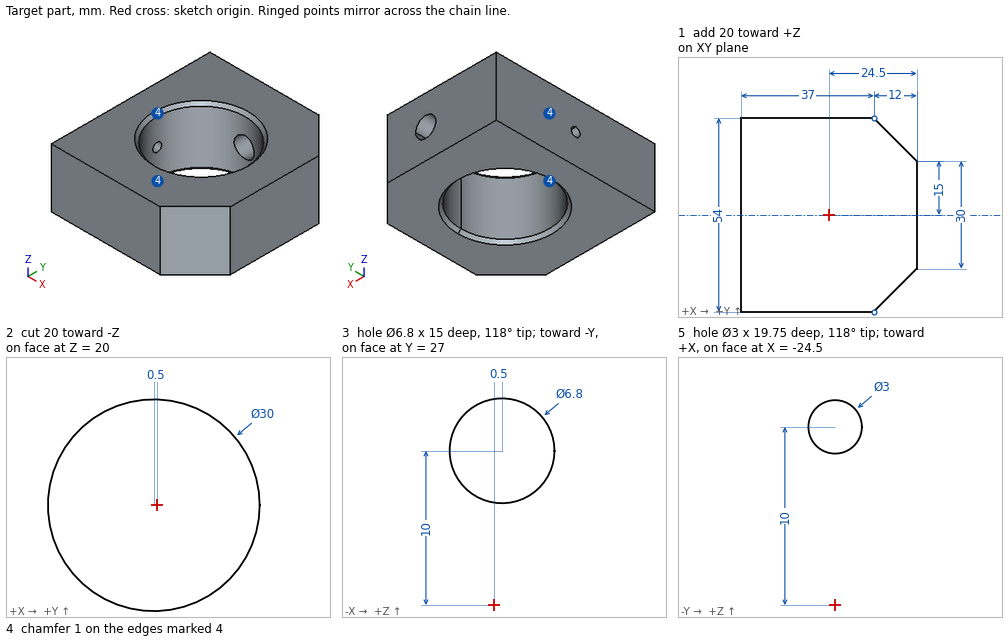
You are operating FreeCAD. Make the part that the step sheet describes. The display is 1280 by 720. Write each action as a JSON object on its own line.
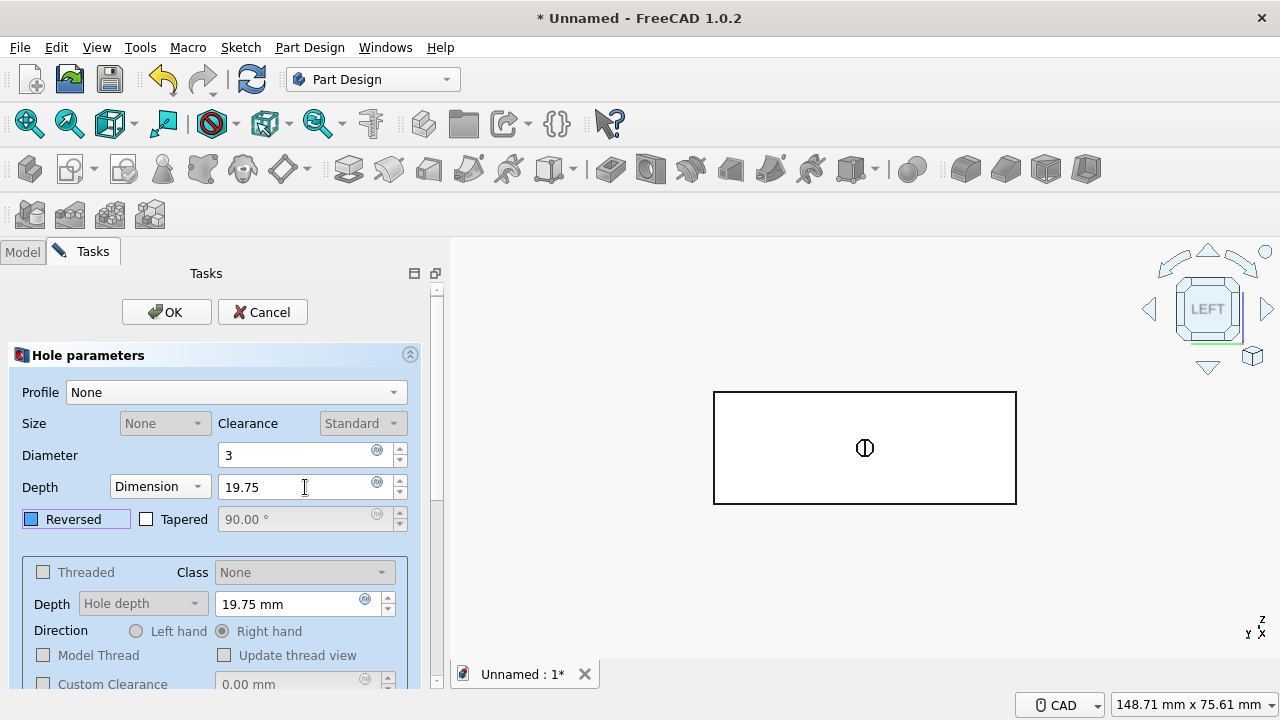
{"action": "left_click", "coordinate": [167, 312]}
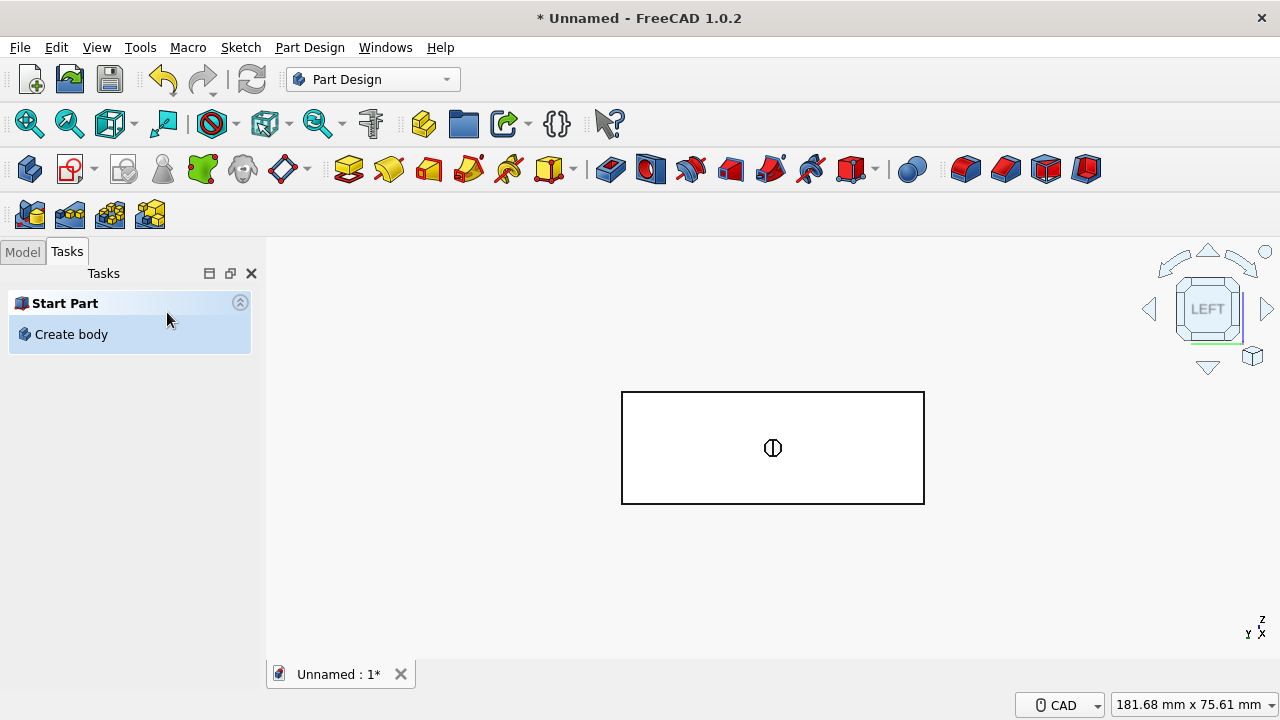
{"action": "key", "text": "0"}